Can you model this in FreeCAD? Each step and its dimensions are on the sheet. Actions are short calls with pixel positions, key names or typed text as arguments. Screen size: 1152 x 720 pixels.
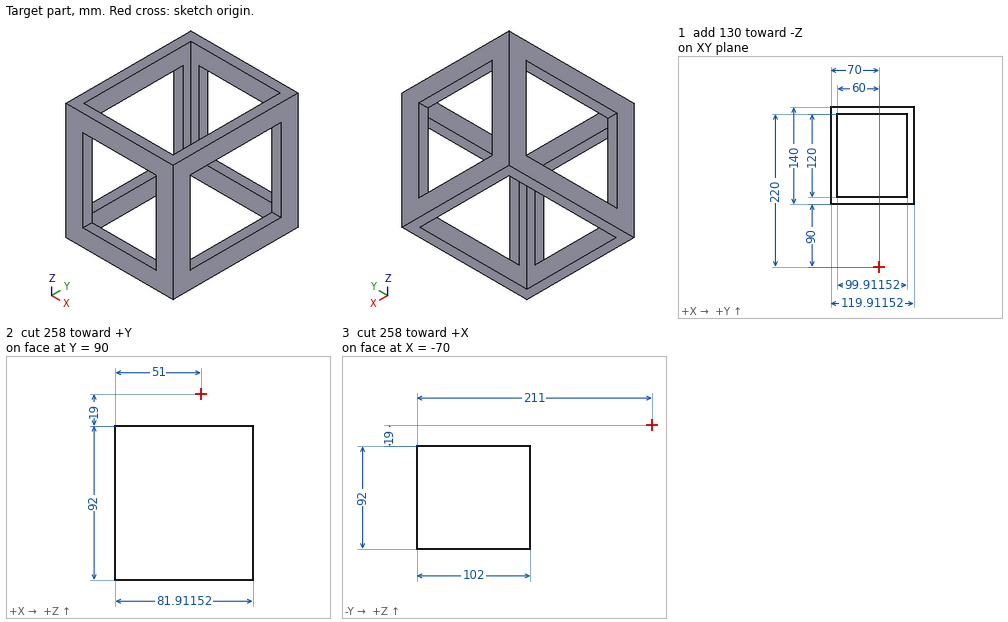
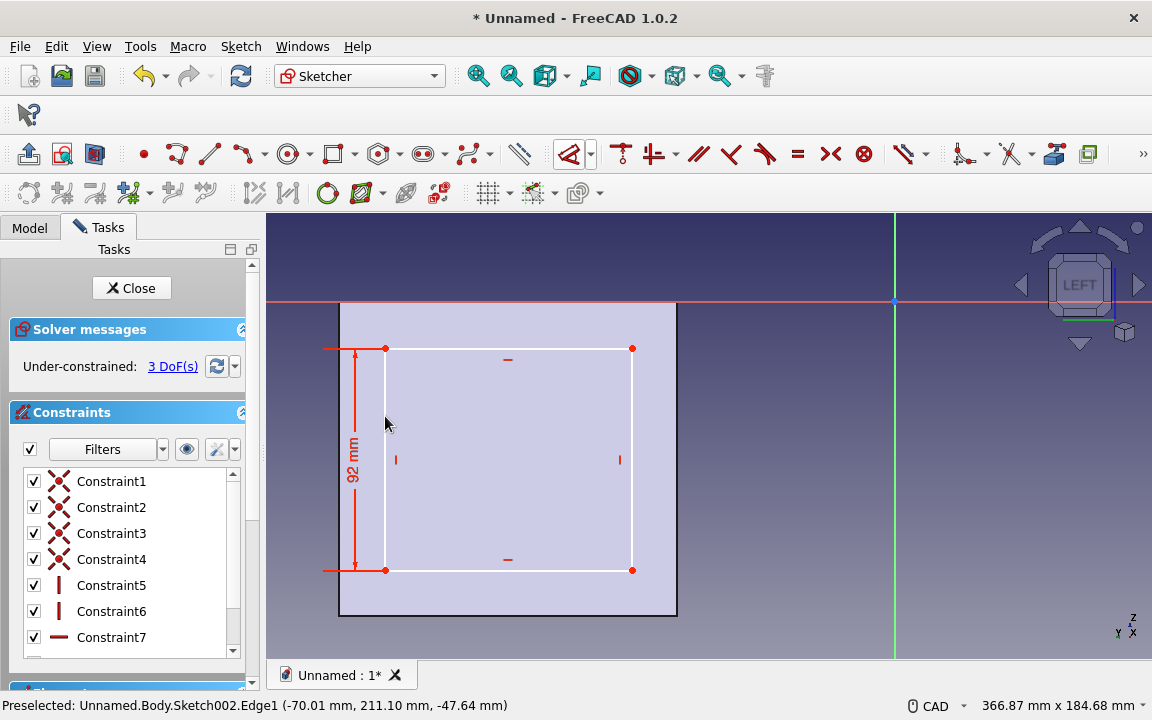
click(459, 571)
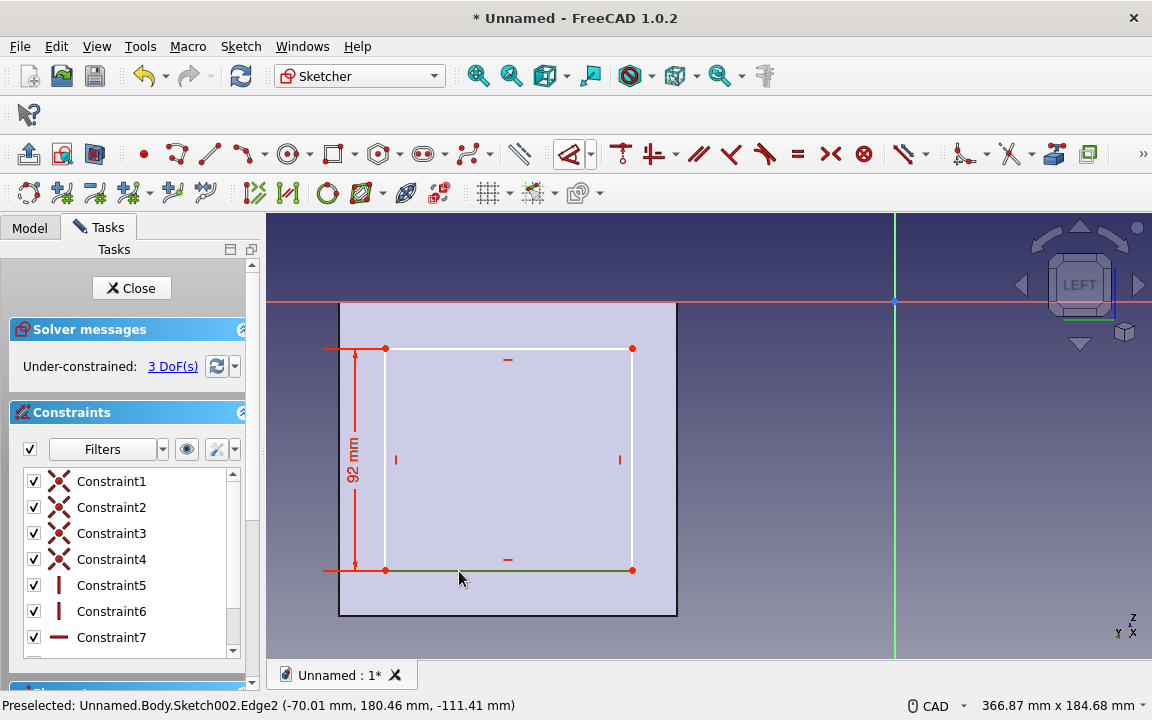
key(l)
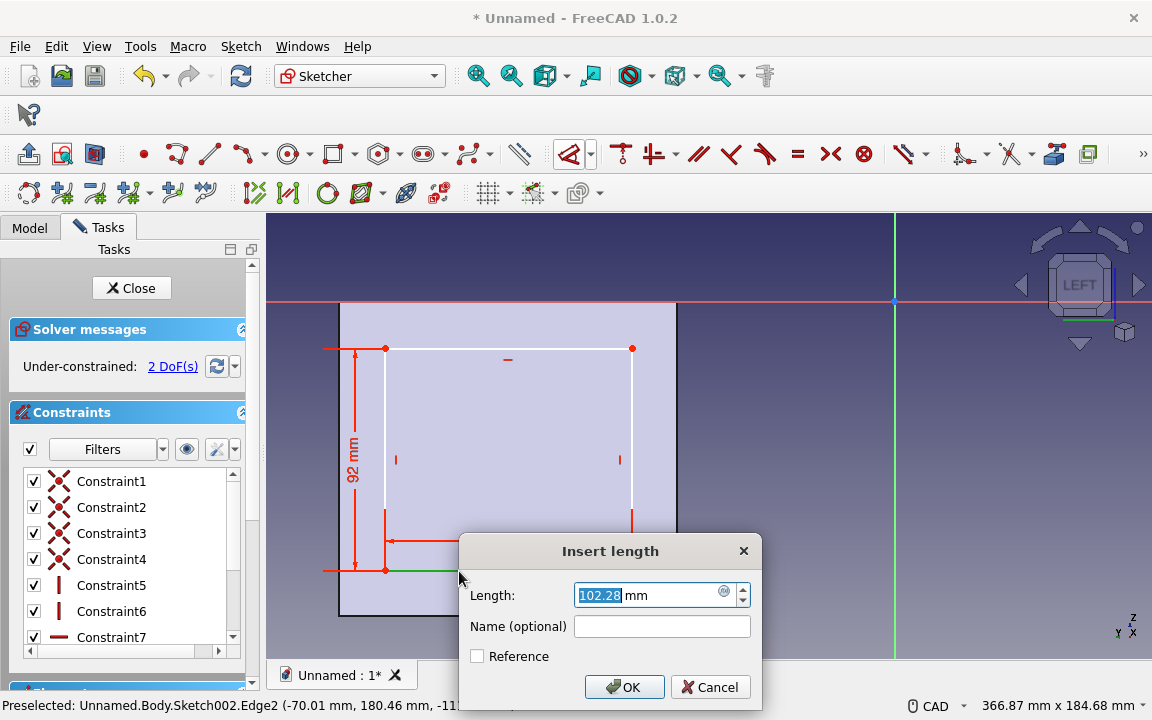
text(102)
key(Return)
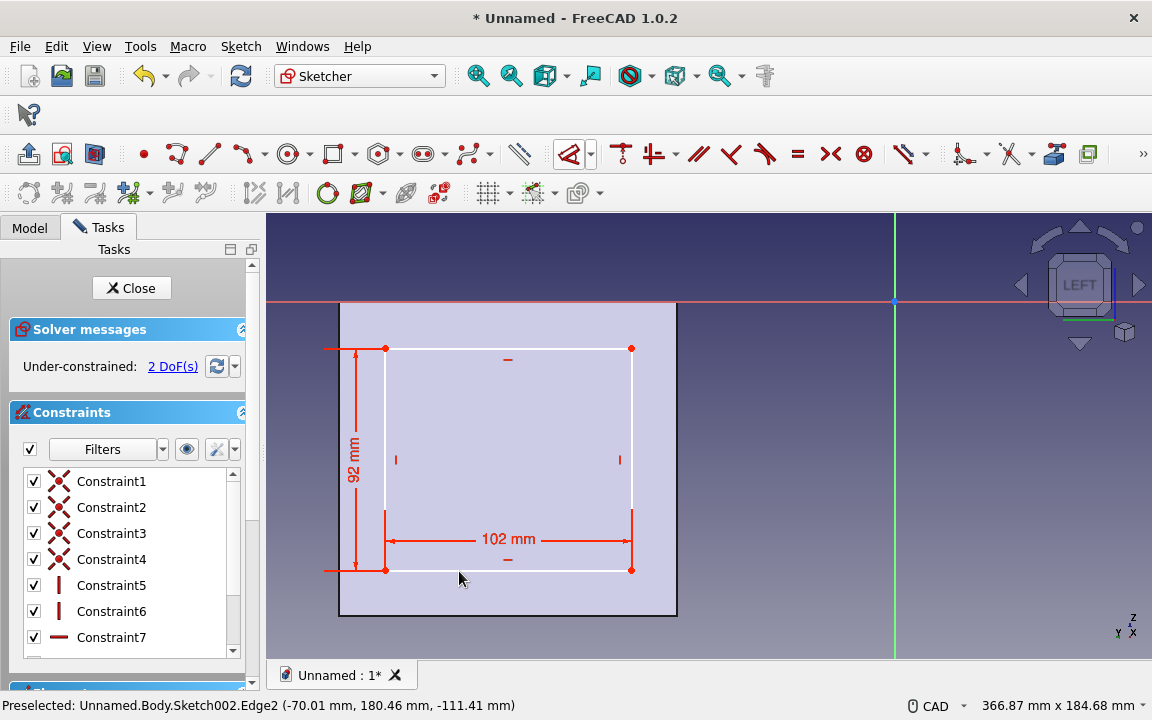
click(385, 349)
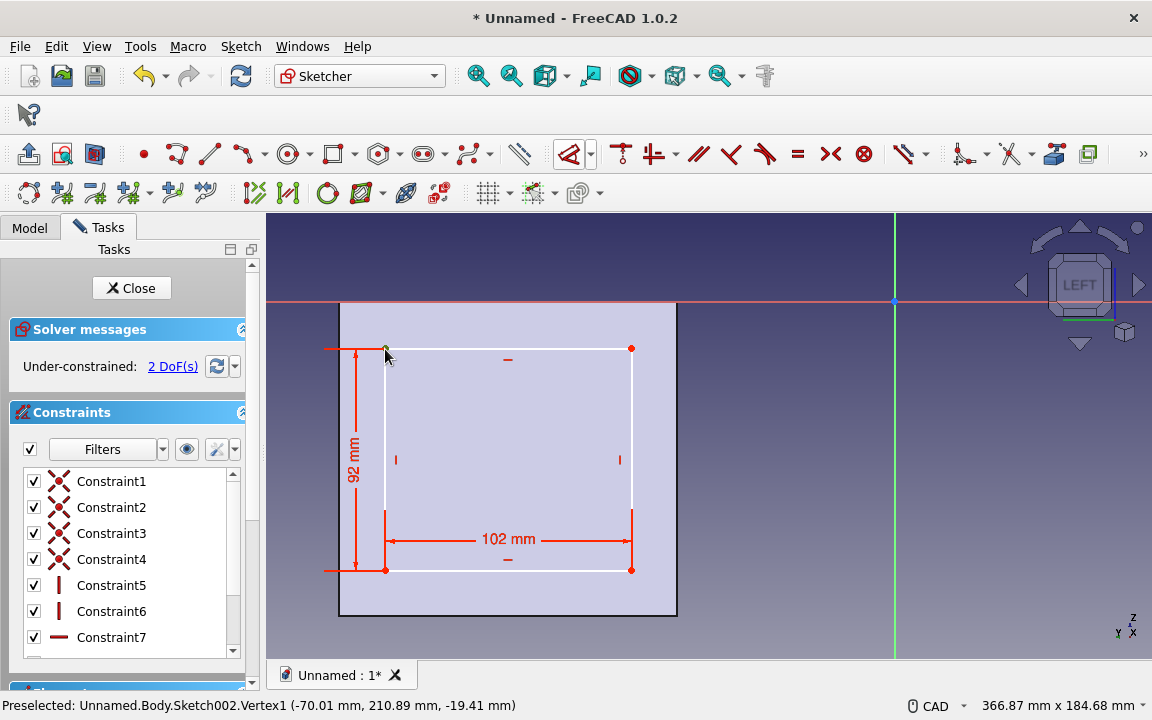
key(i)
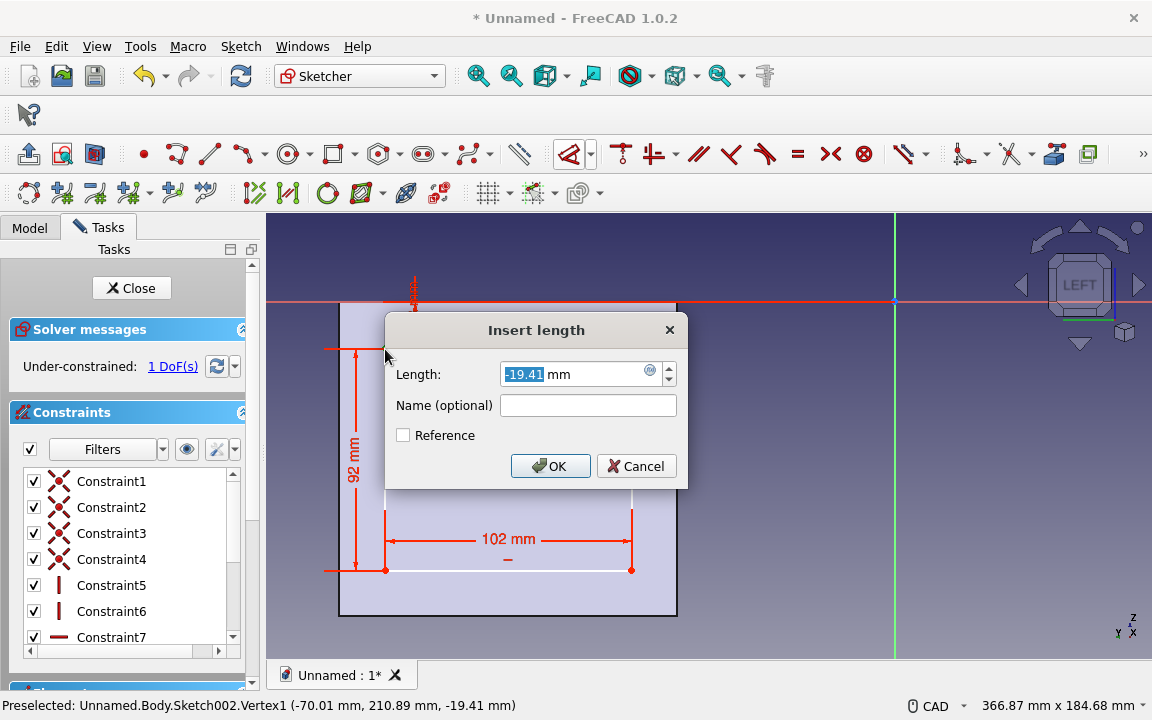
text(-19)
key(Return)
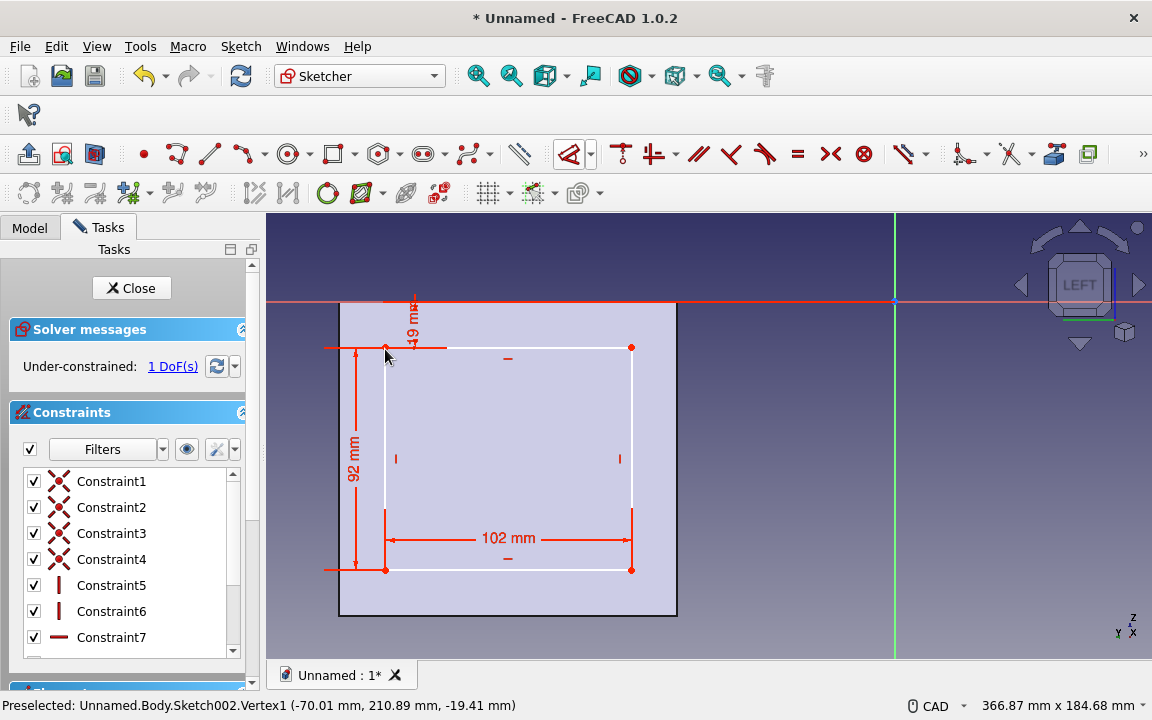
click(385, 348)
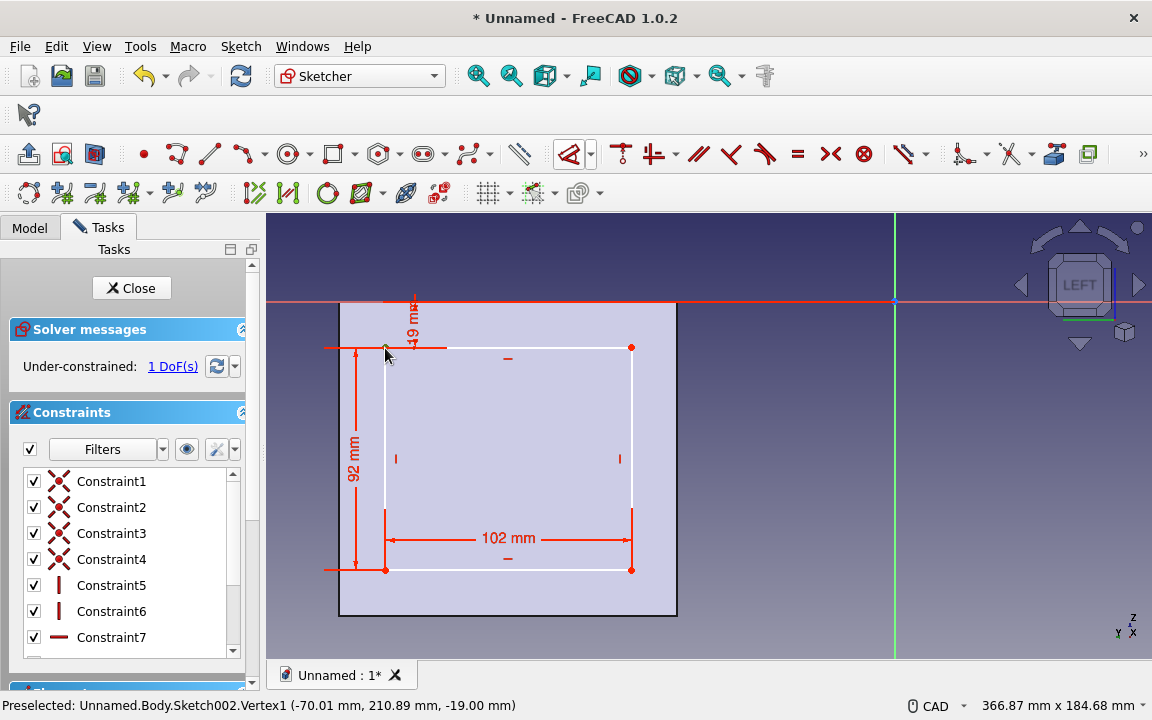
key(l)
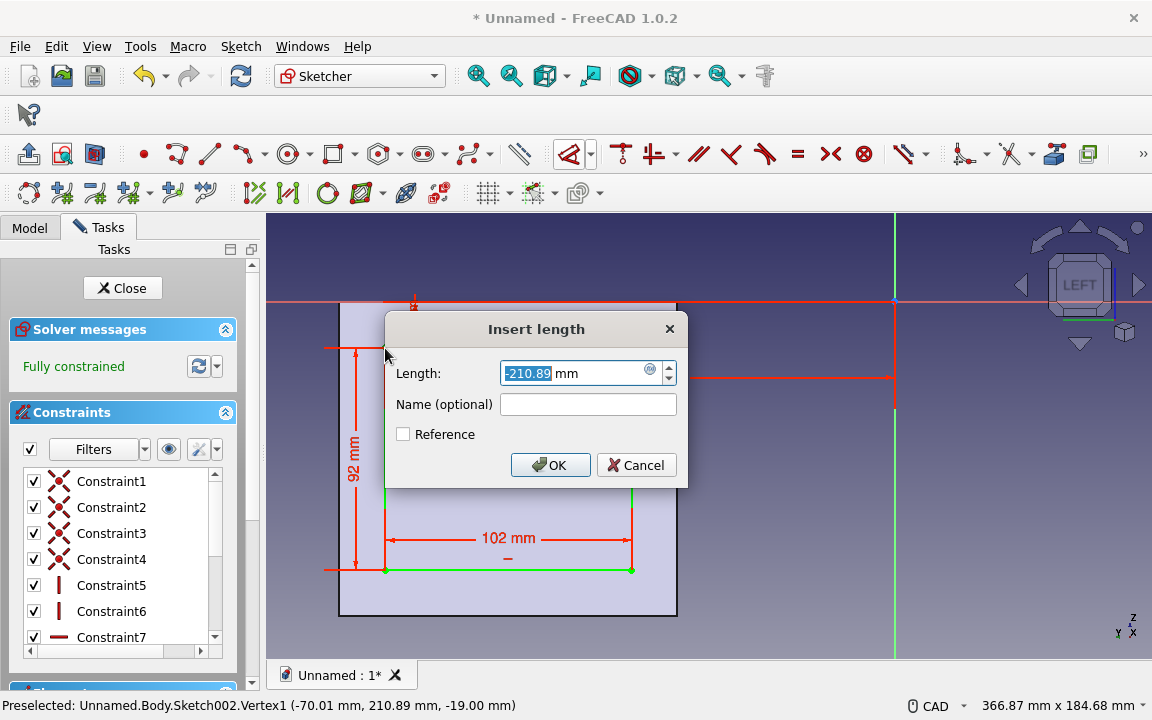
text(-211)
key(Return)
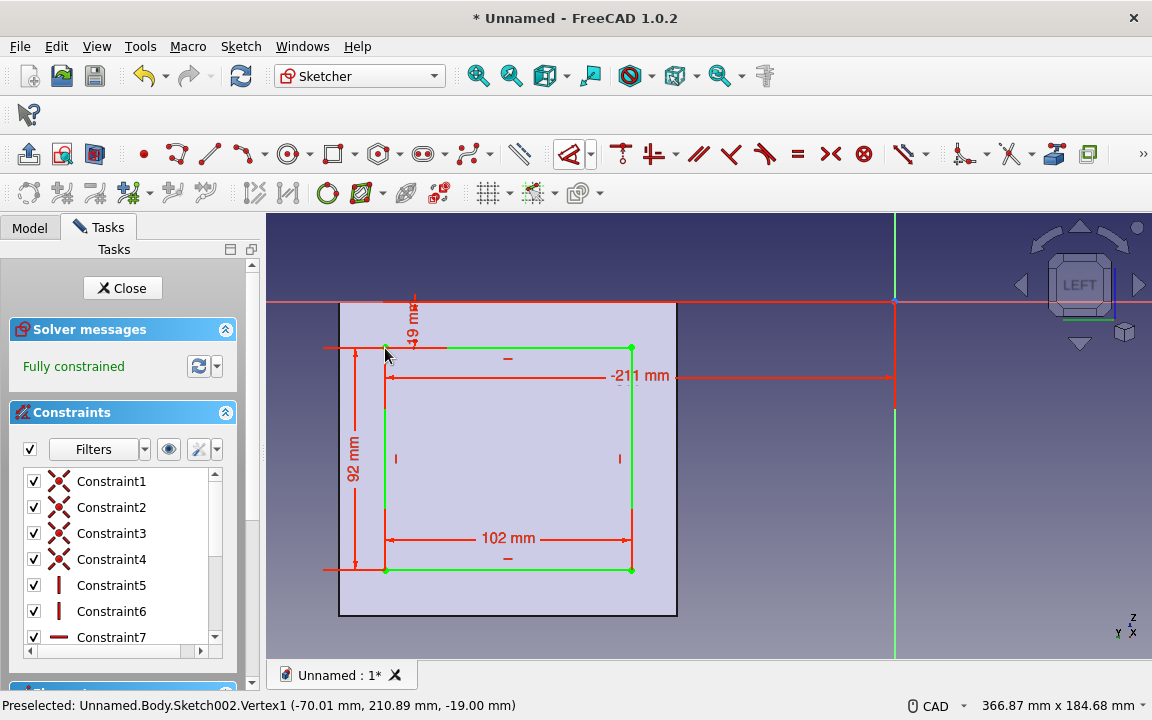
click(123, 288)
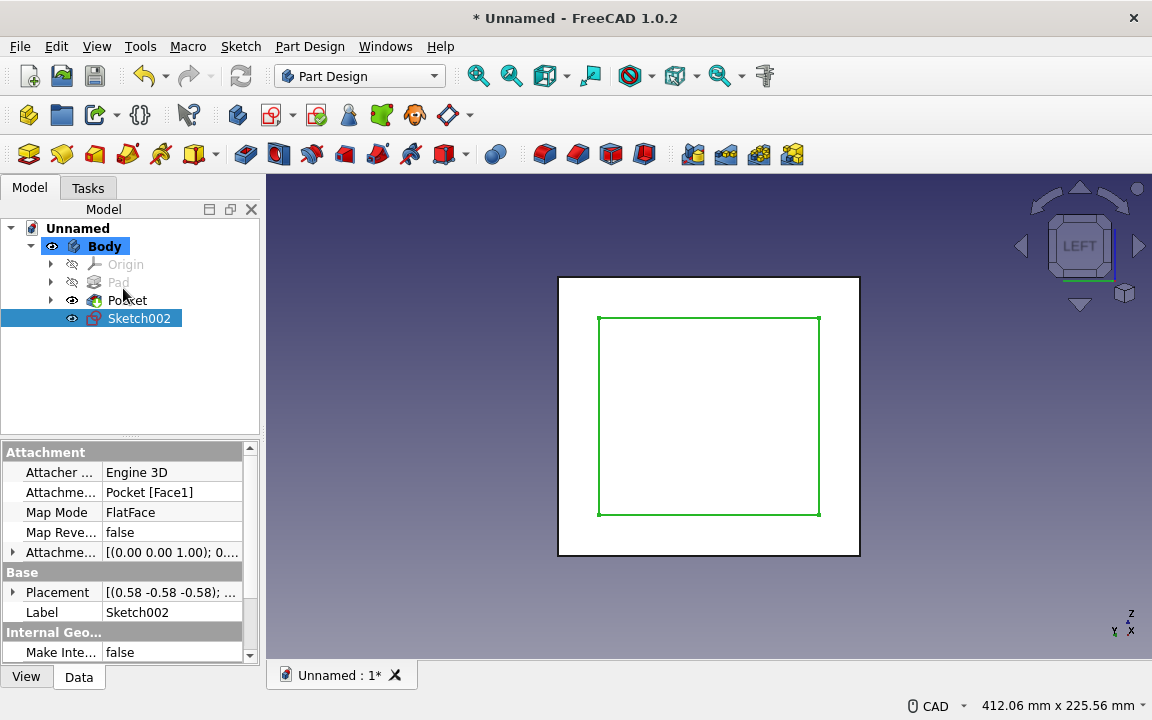
click(246, 154)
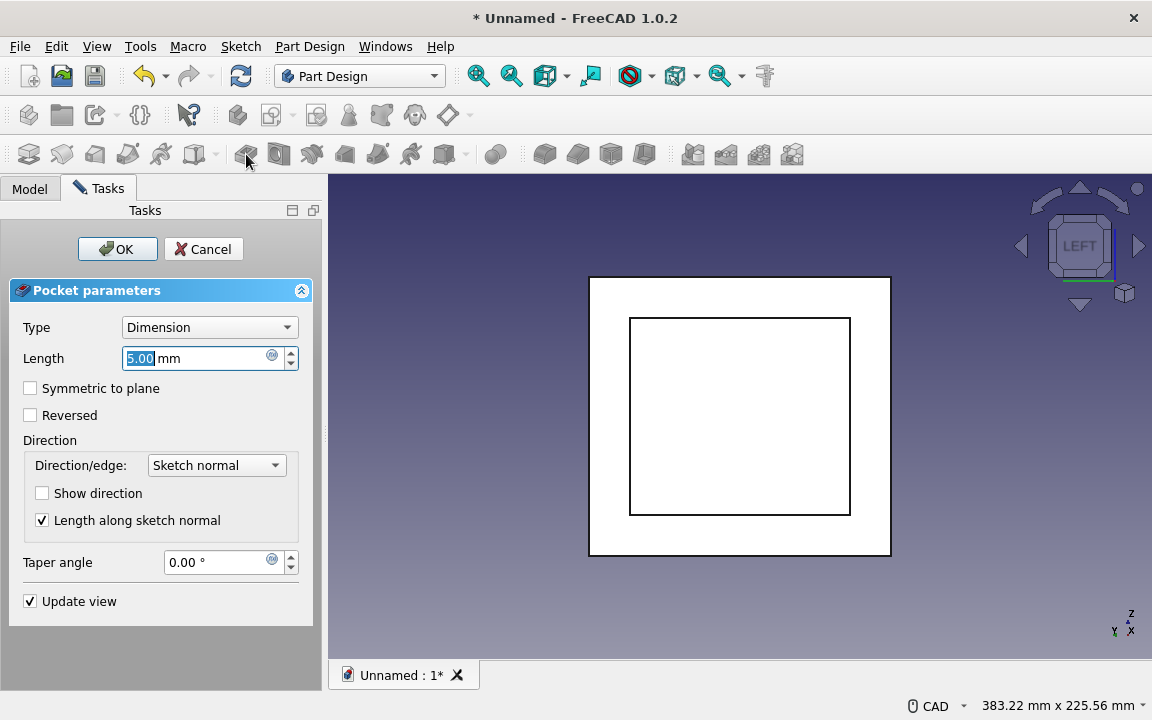
text(258)
key(Tab)